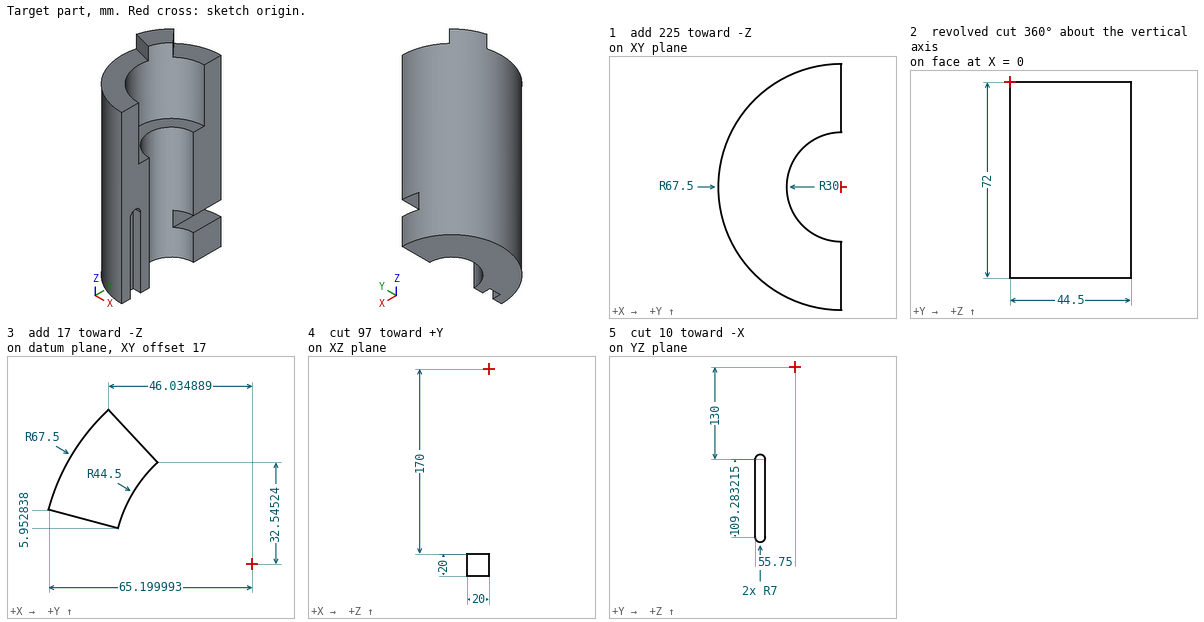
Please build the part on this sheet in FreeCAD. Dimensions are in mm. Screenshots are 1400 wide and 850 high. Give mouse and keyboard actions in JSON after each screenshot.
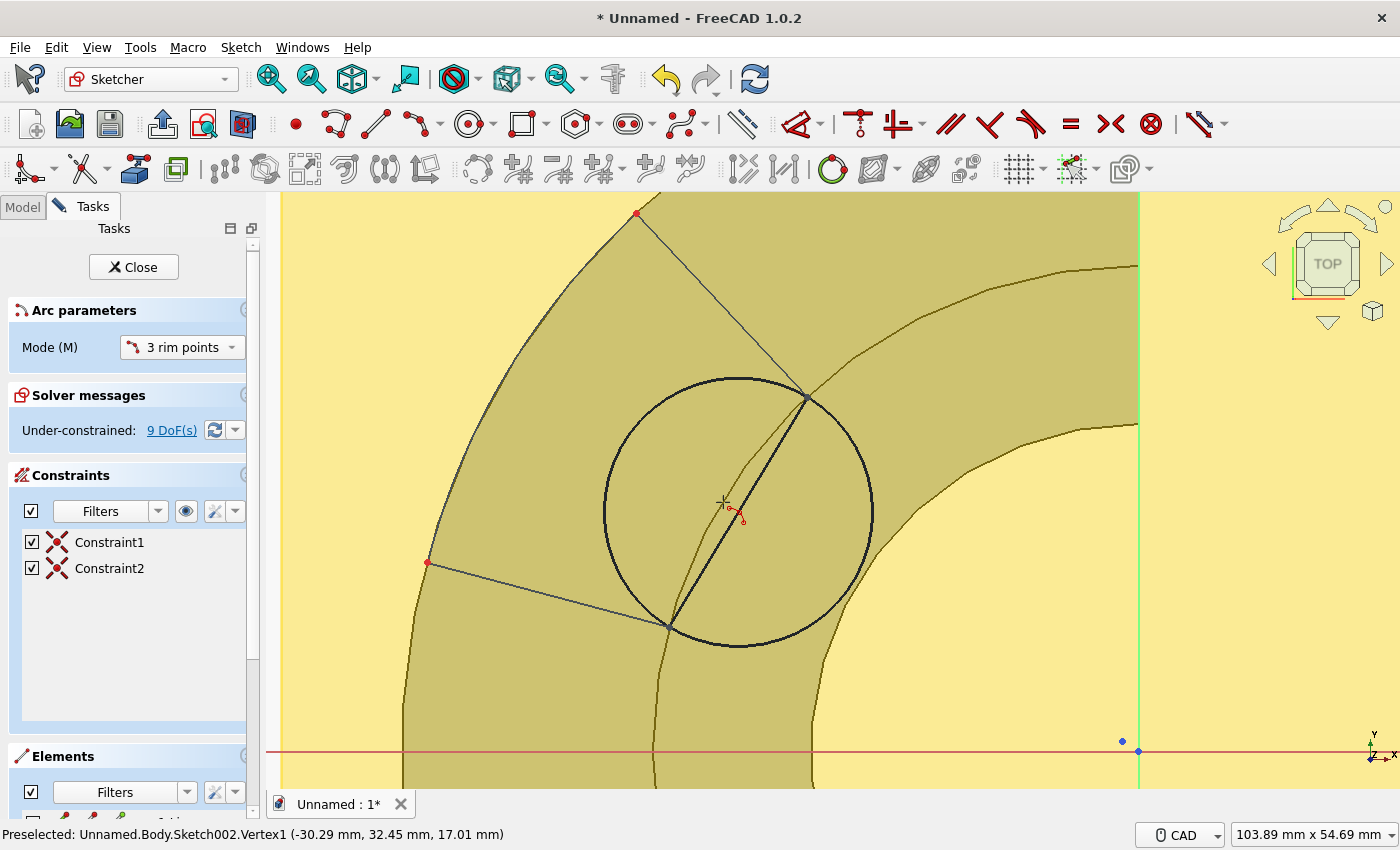
{"action": "left_click", "coordinate": [722, 501]}
{"action": "key", "text": "Escape"}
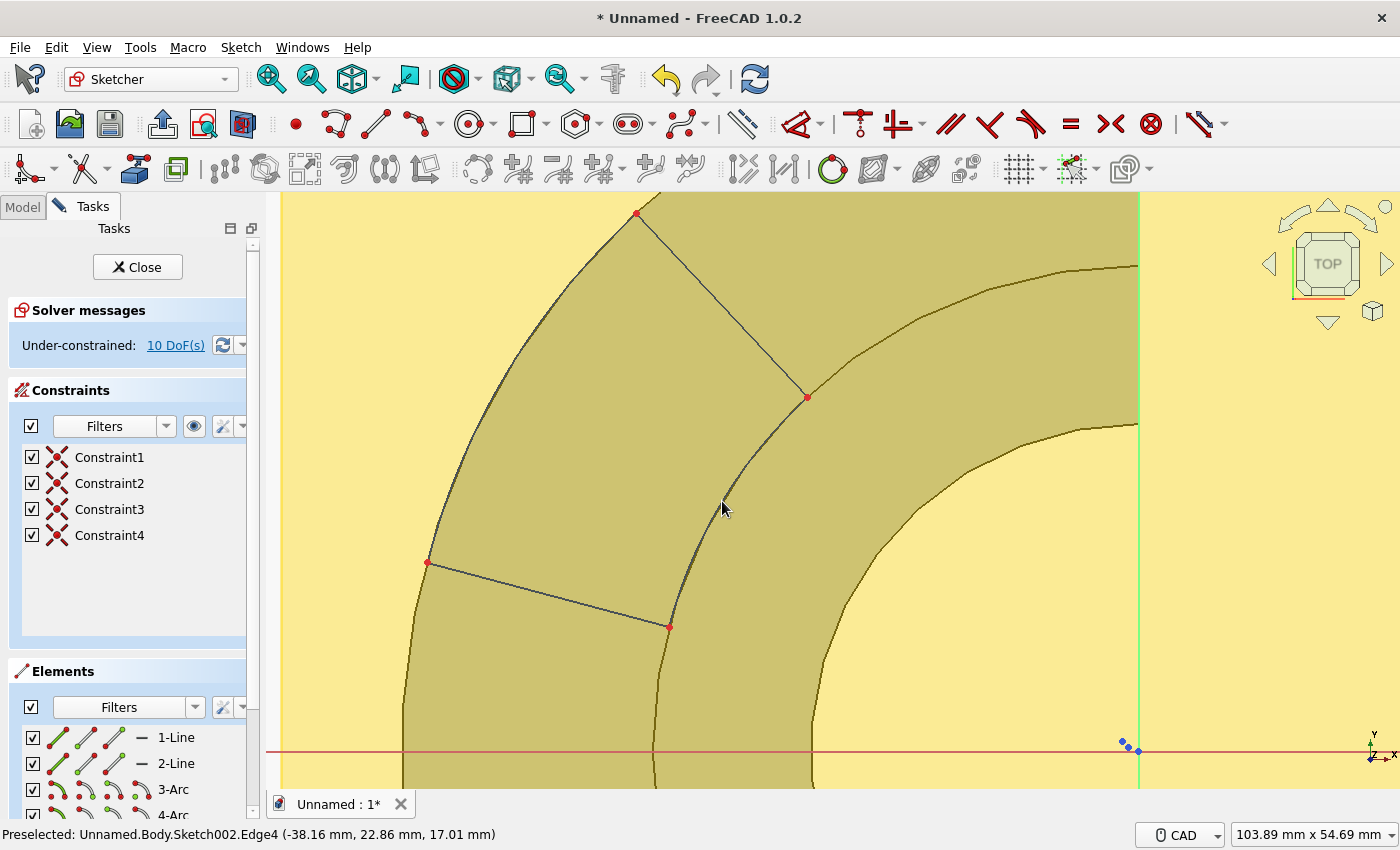
{"action": "left_click", "coordinate": [553, 305]}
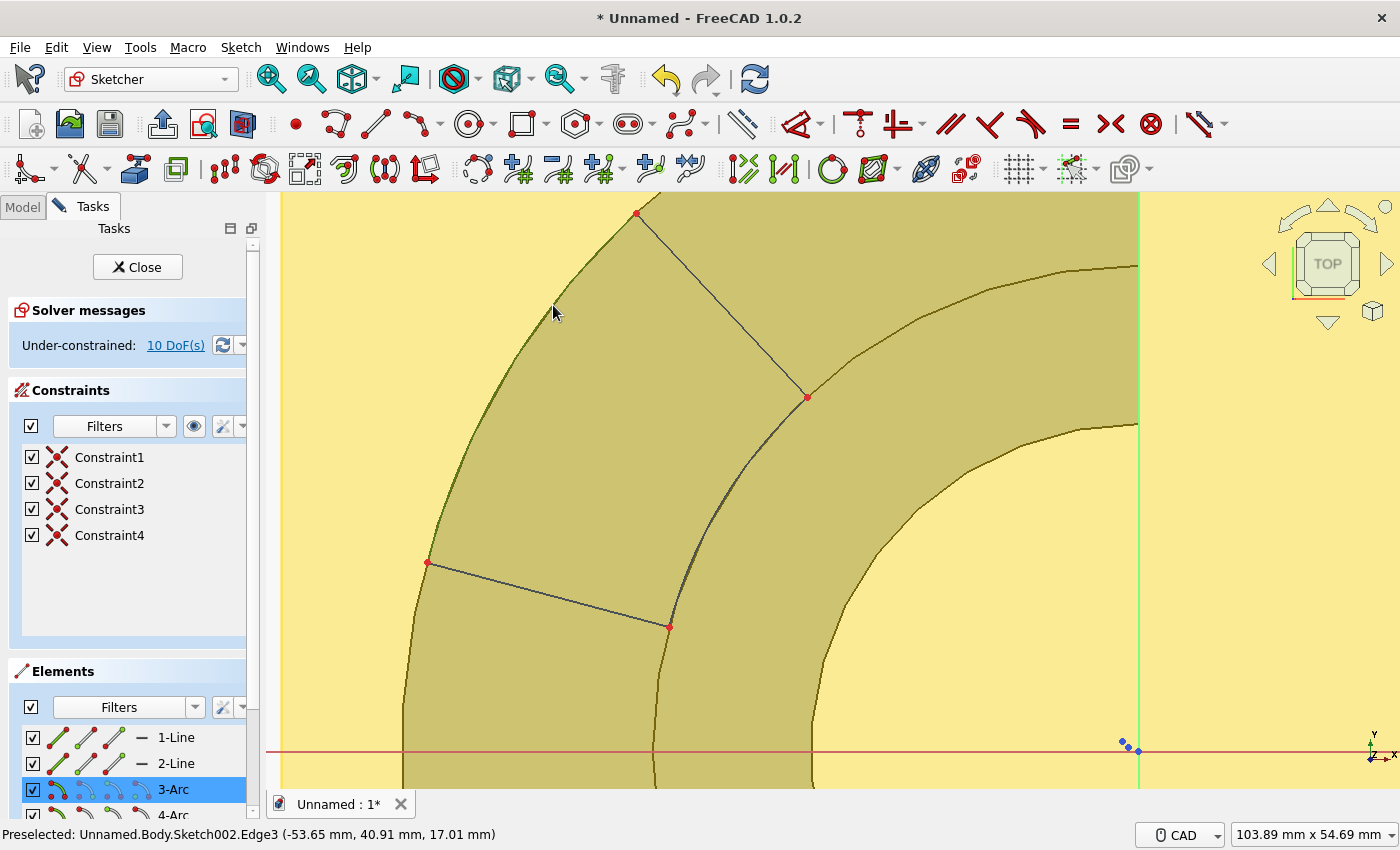
{"action": "left_click", "coordinate": [753, 457]}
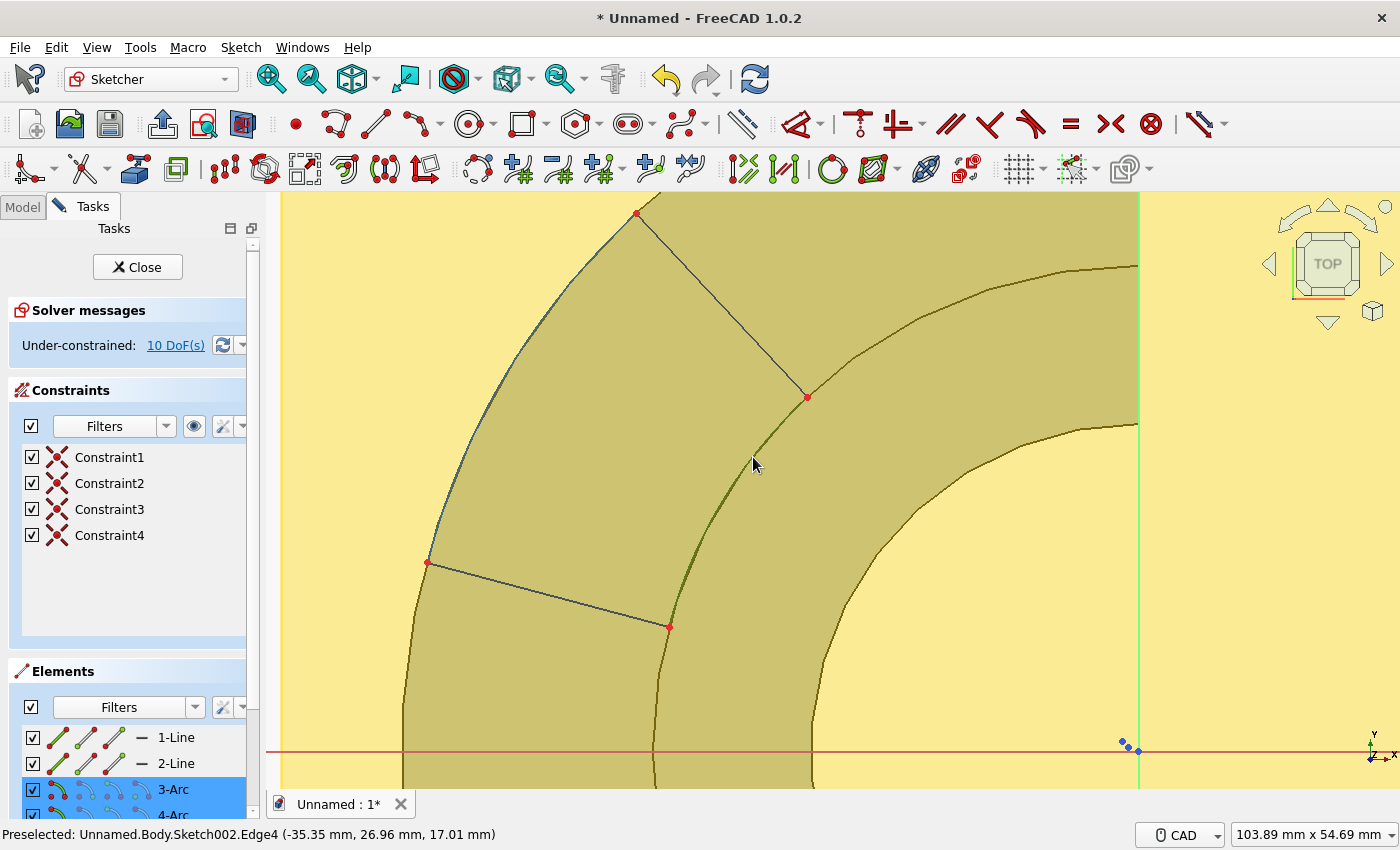
{"action": "left_click", "coordinate": [858, 124]}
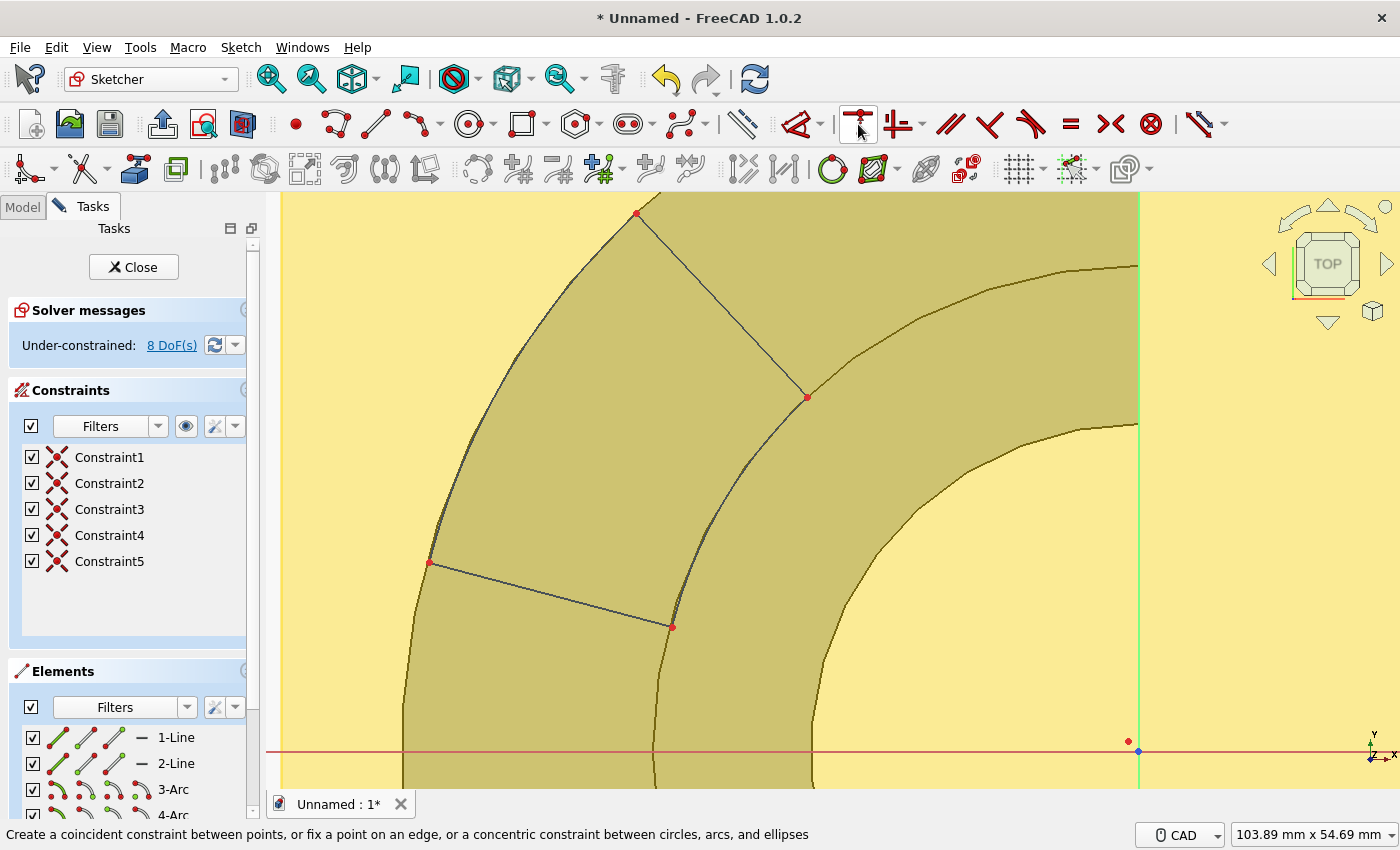
{"action": "left_click_drag", "start_coordinate": [1118, 732], "coordinate": [1149, 762]}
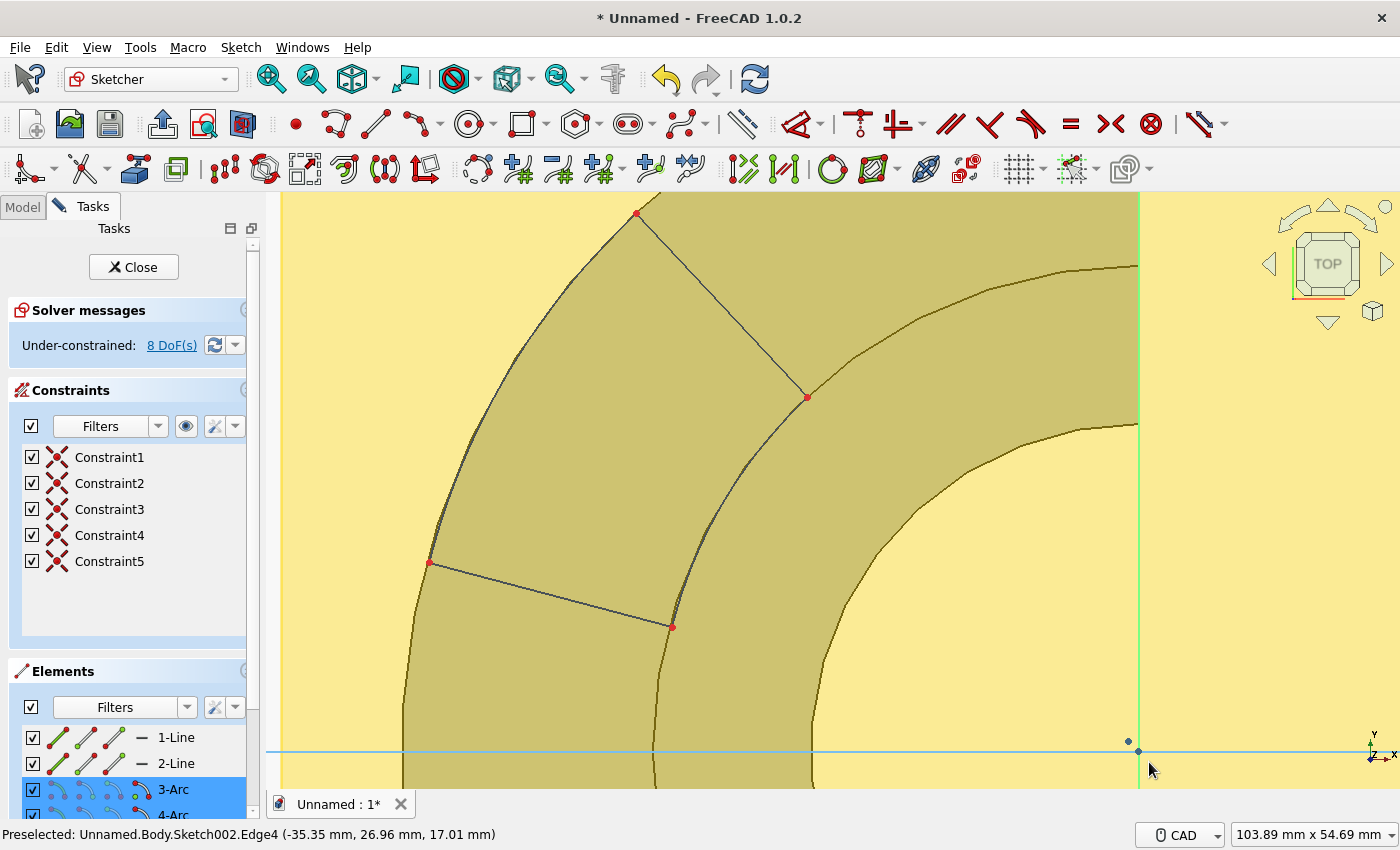
{"action": "key", "text": "c"}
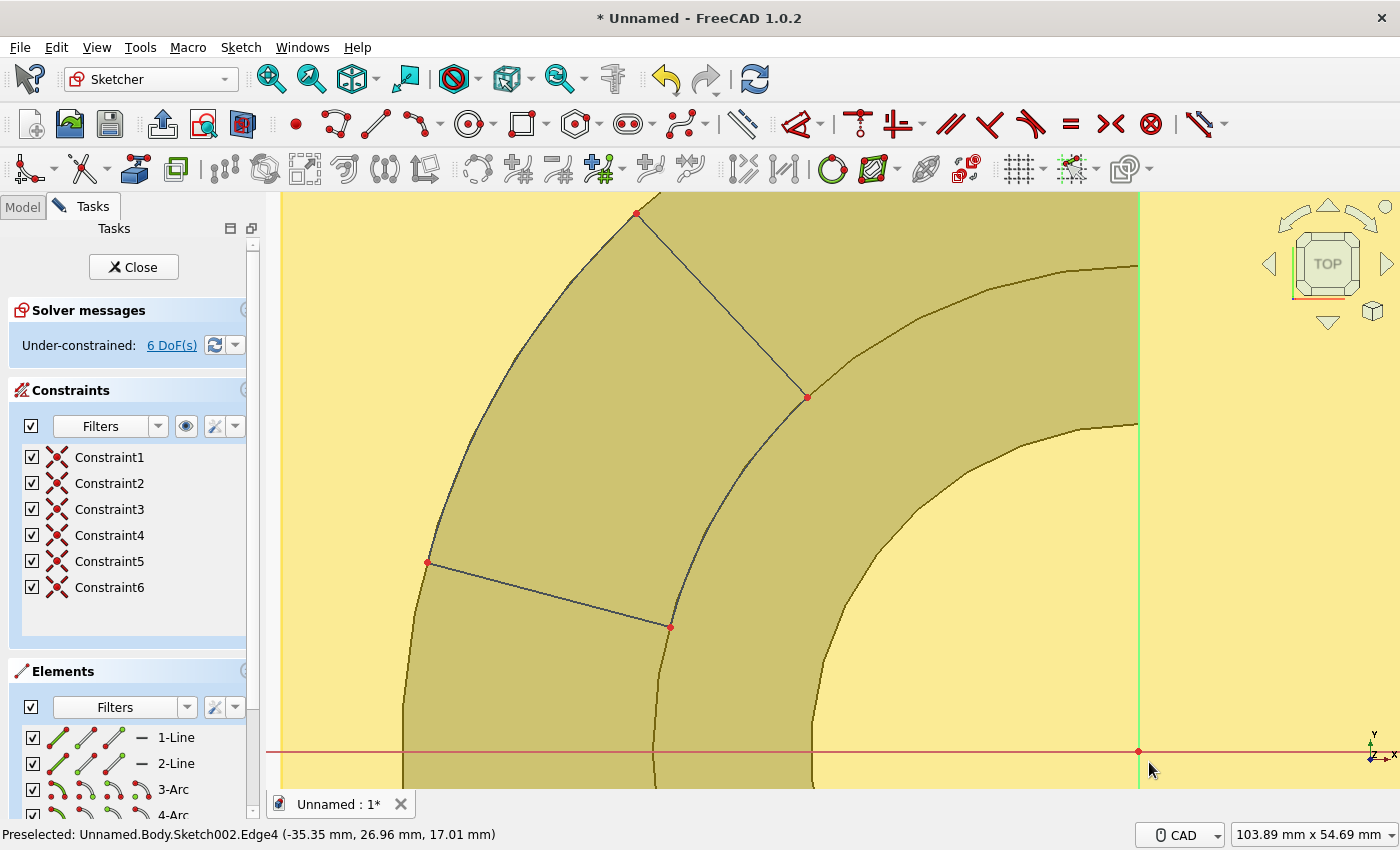
{"action": "left_click", "coordinate": [553, 305]}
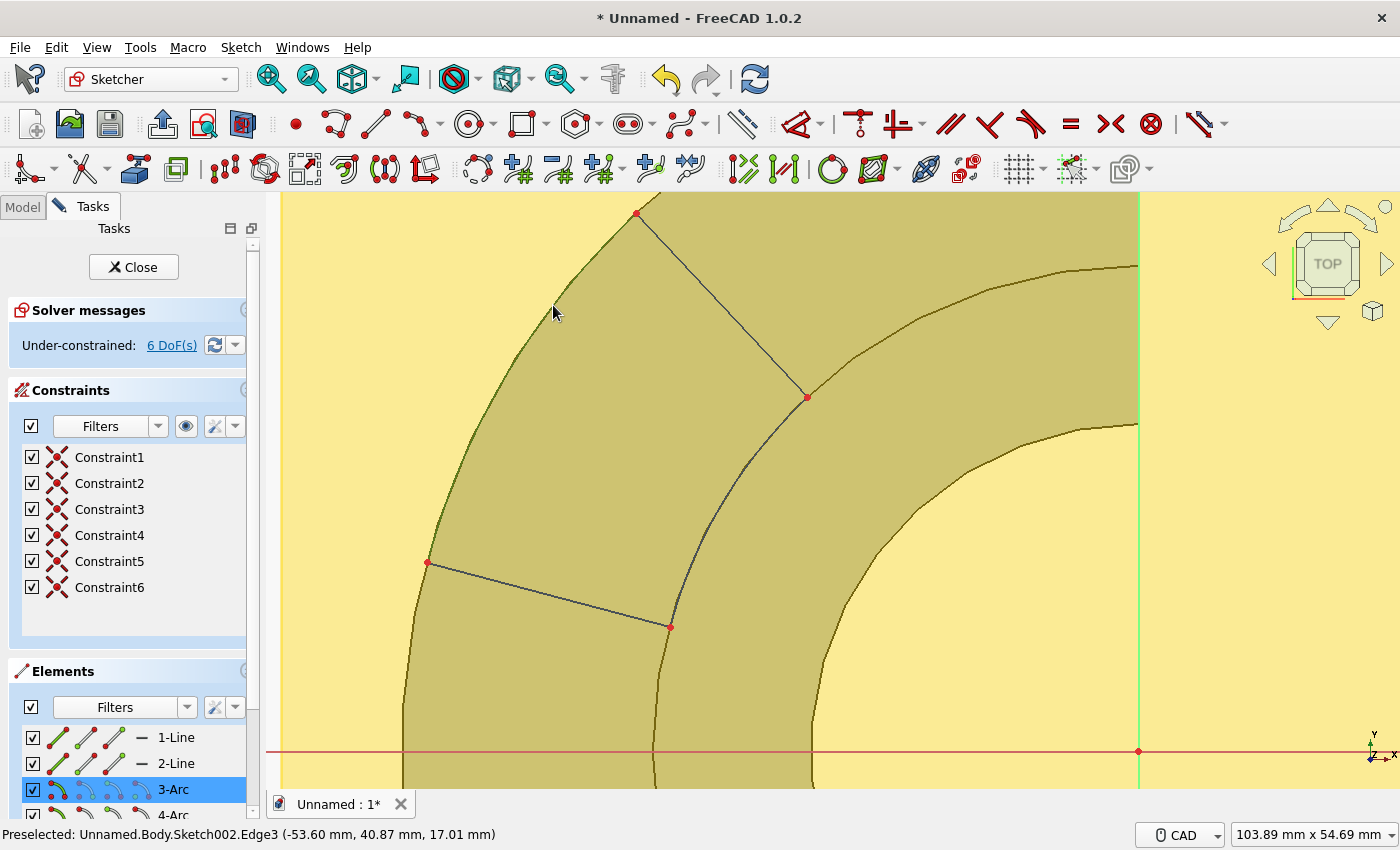
{"action": "key", "text": "k r"}